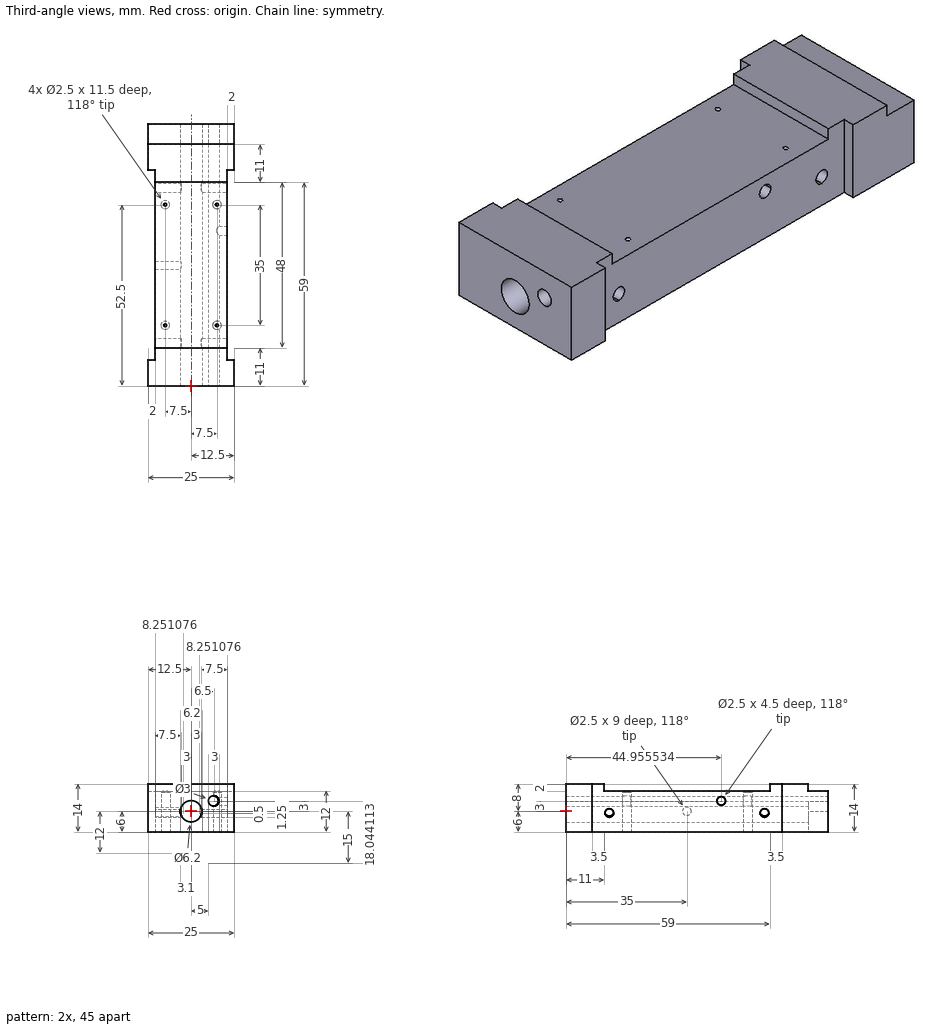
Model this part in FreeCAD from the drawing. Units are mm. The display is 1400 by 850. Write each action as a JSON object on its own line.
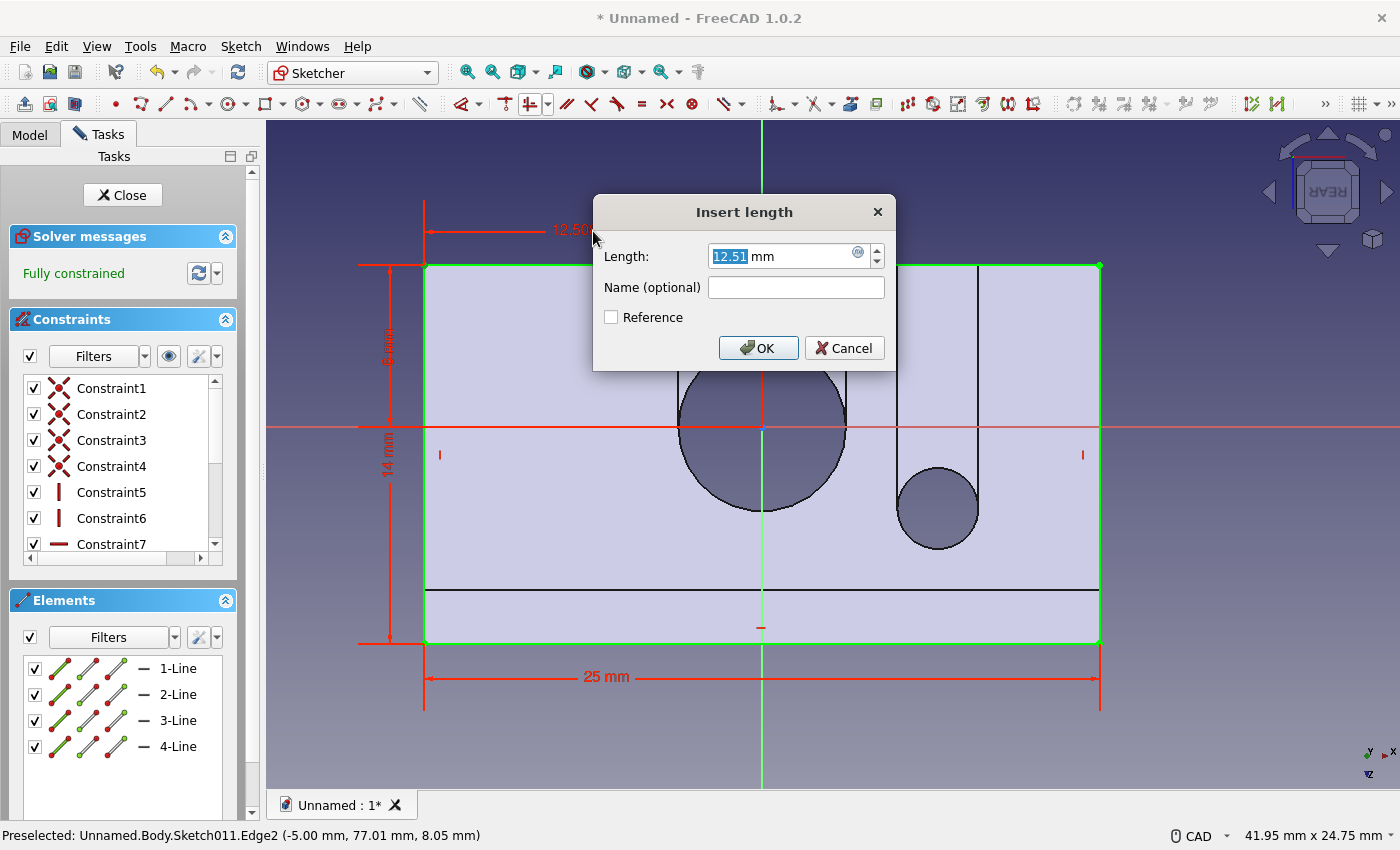
{"action": "type", "text": "12.5"}
{"action": "key", "text": "Return"}
{"action": "key", "text": "Escape"}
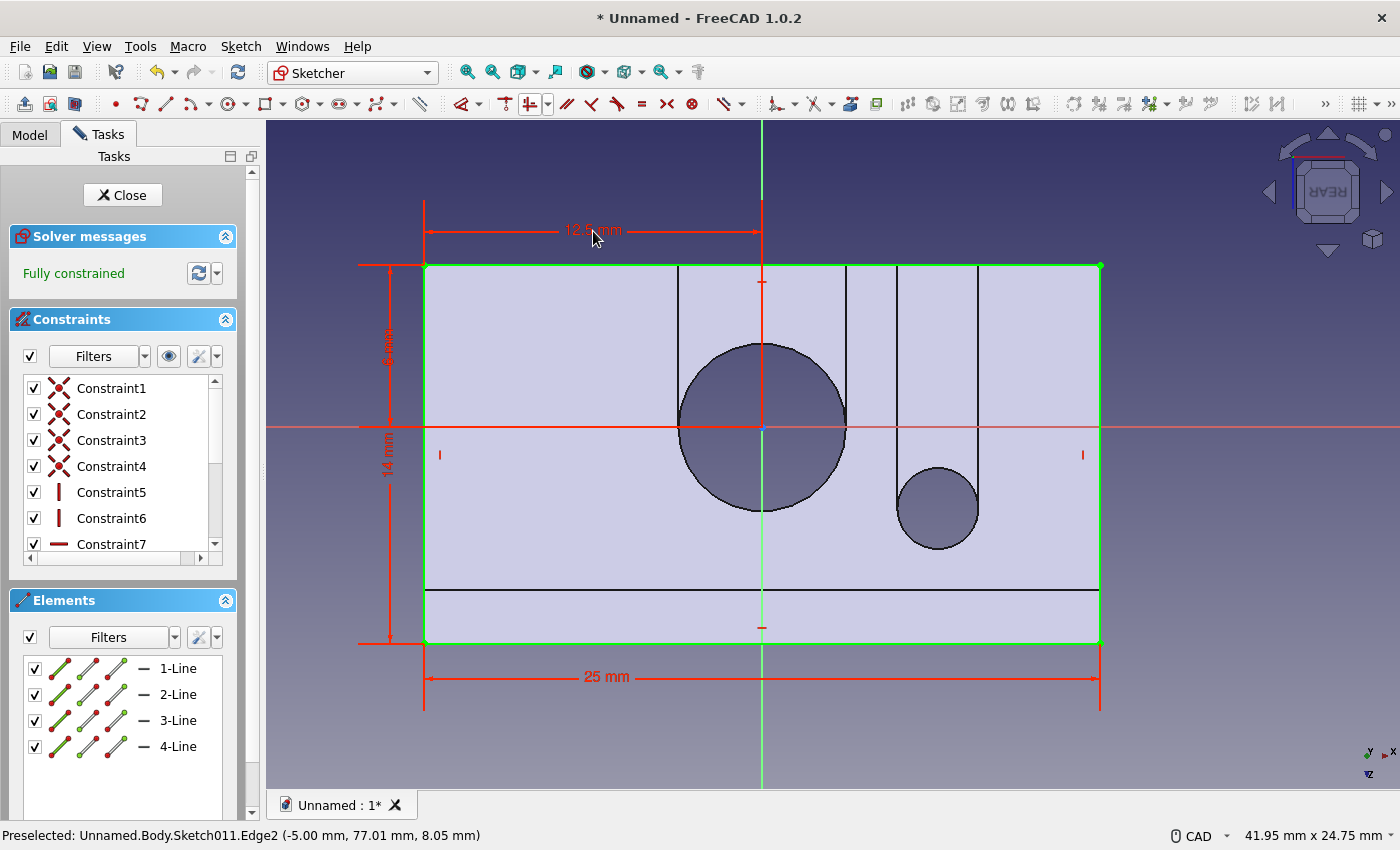
{"action": "left_click", "coordinate": [123, 195]}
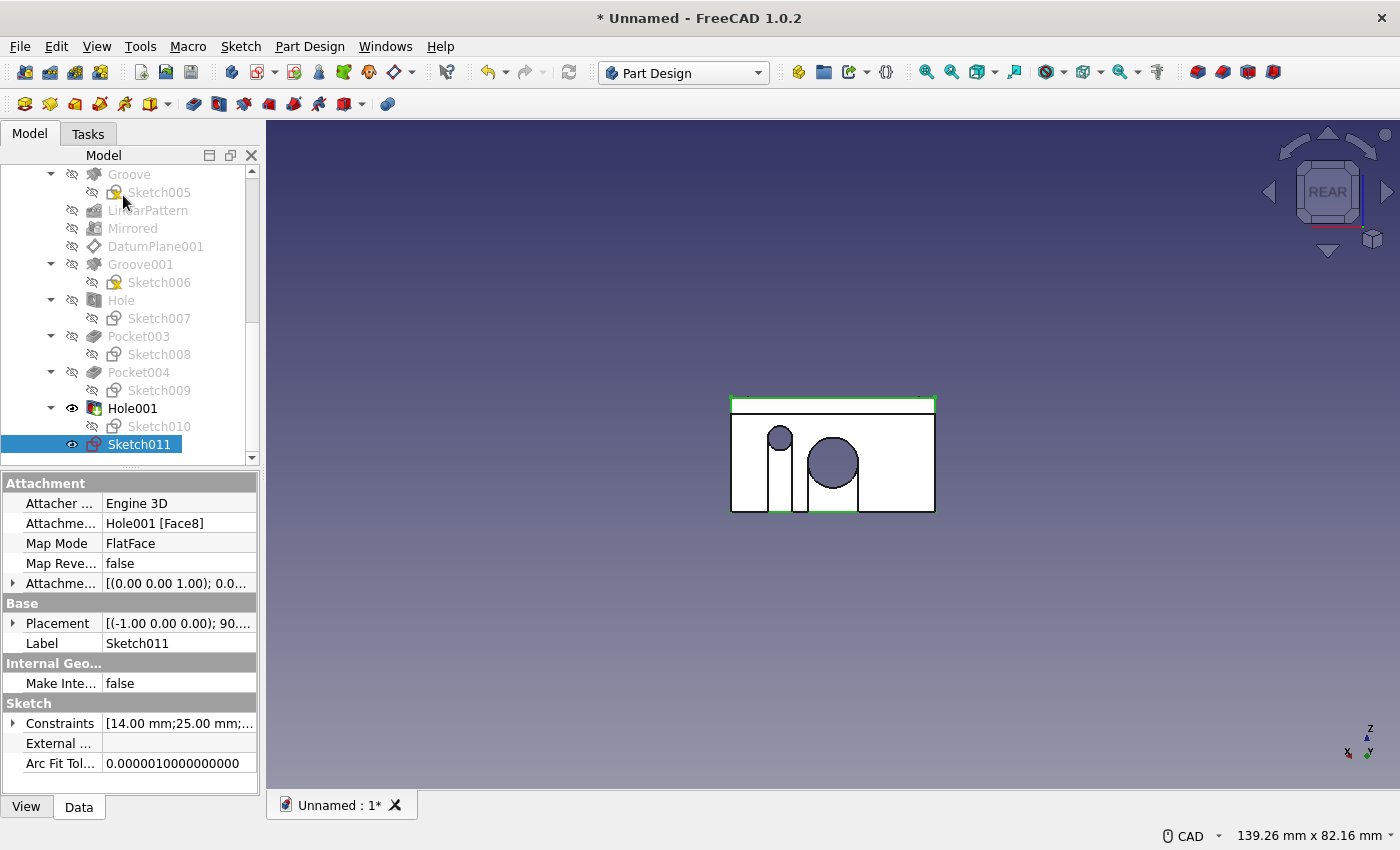
{"action": "left_click", "coordinate": [194, 104]}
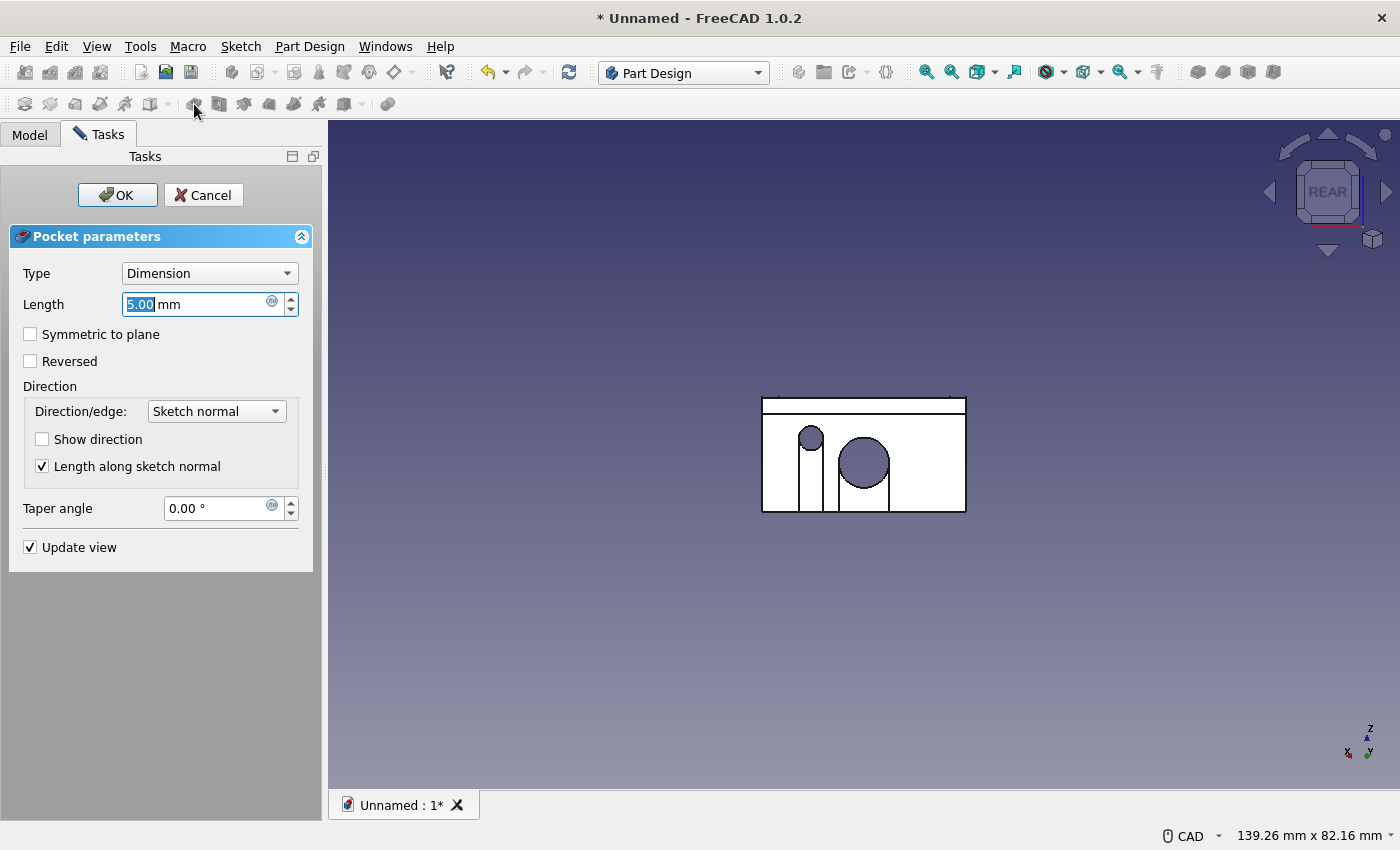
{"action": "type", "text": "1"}
{"action": "key", "text": "Tab"}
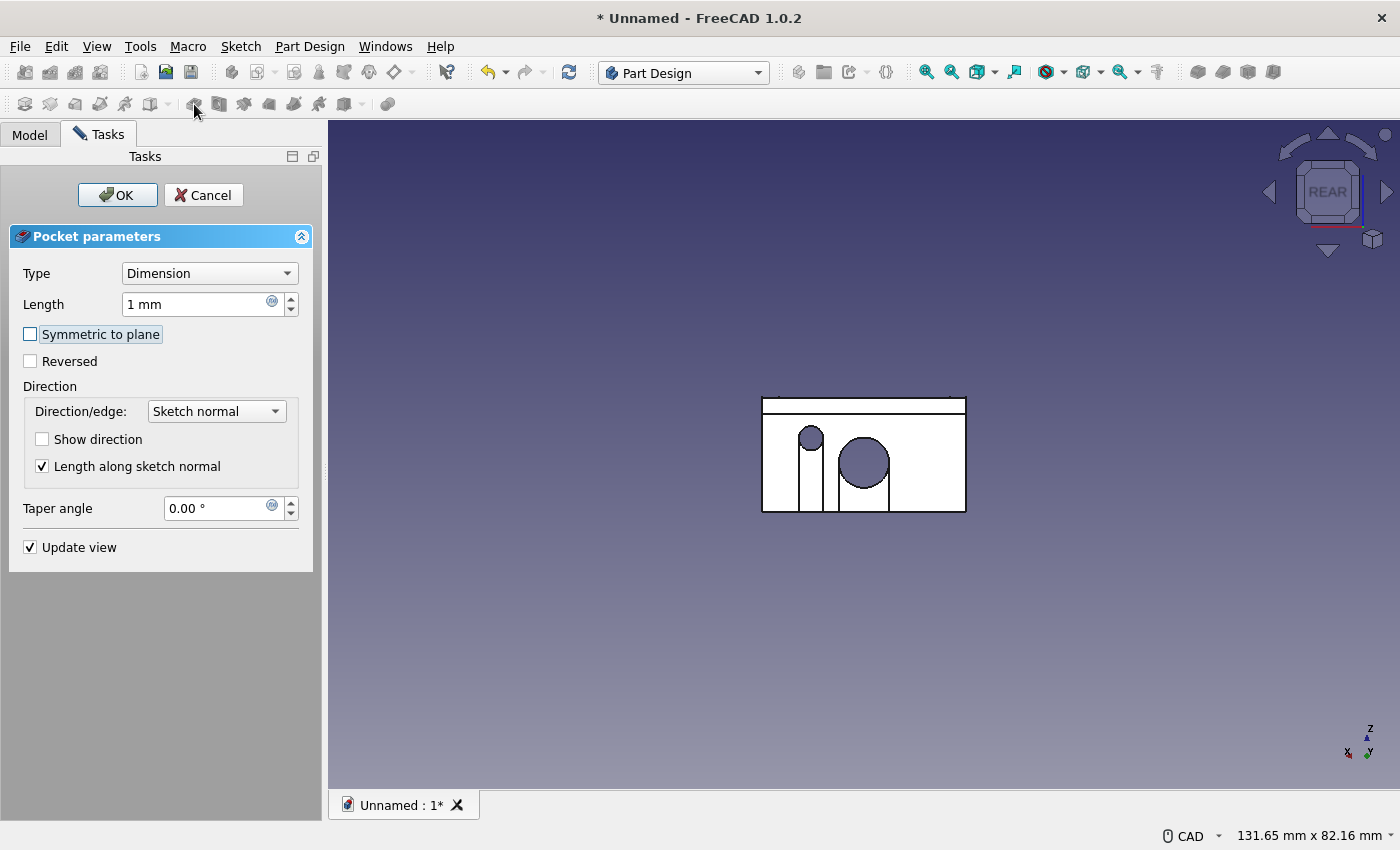
{"action": "left_click", "coordinate": [118, 195]}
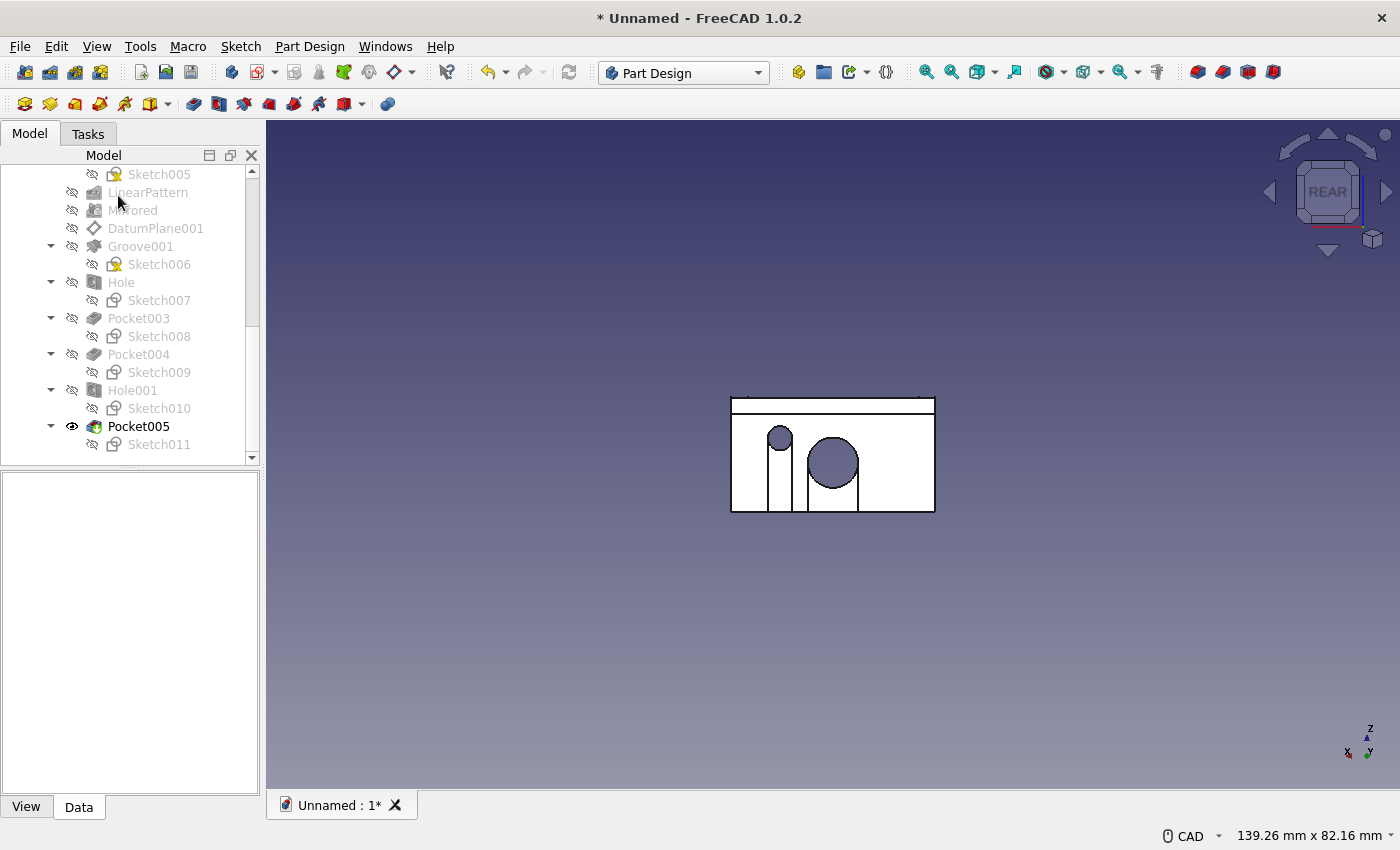
{"action": "left_click", "coordinate": [927, 72]}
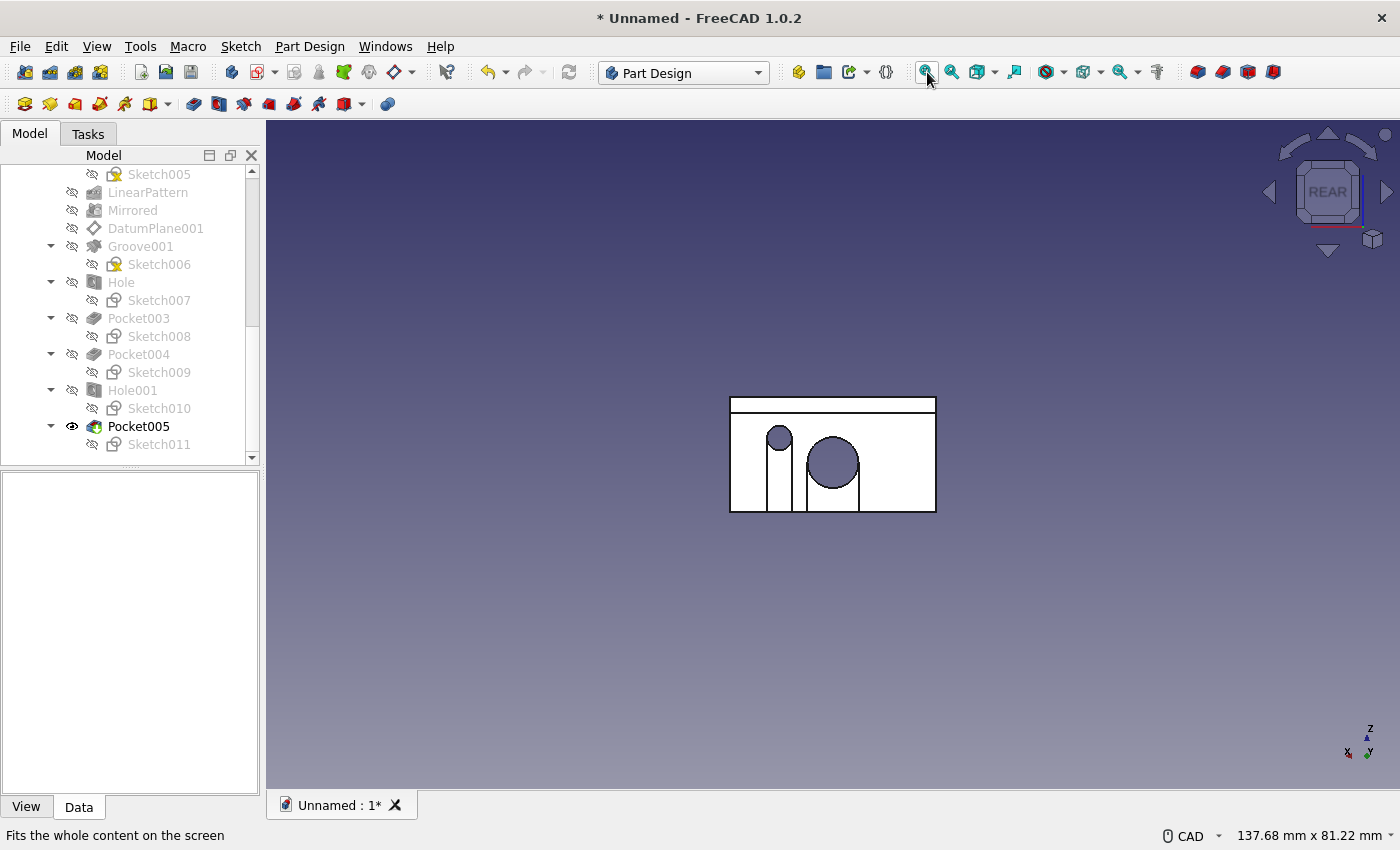
{"action": "key", "text": "6"}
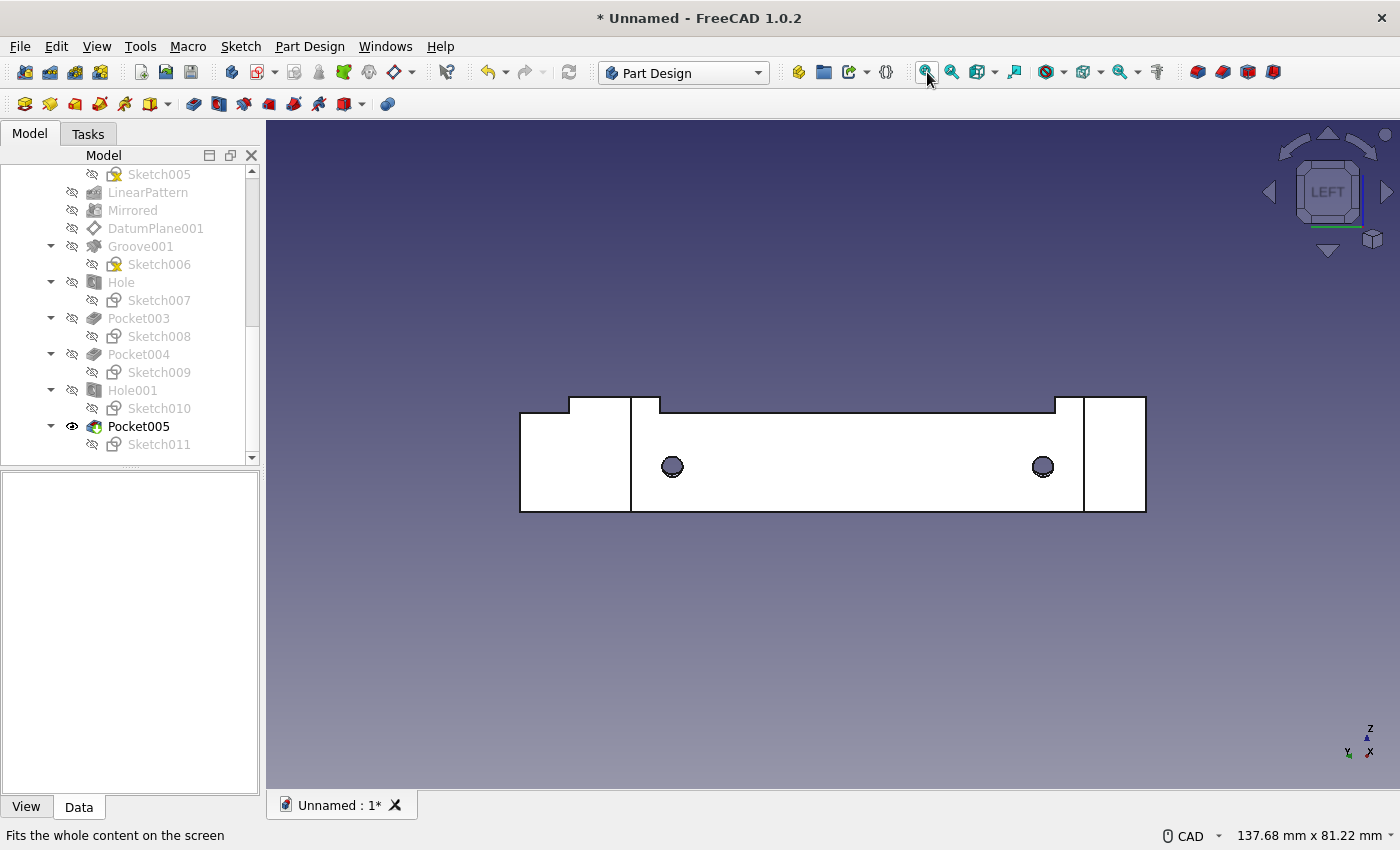
{"action": "left_click", "coordinate": [987, 454]}